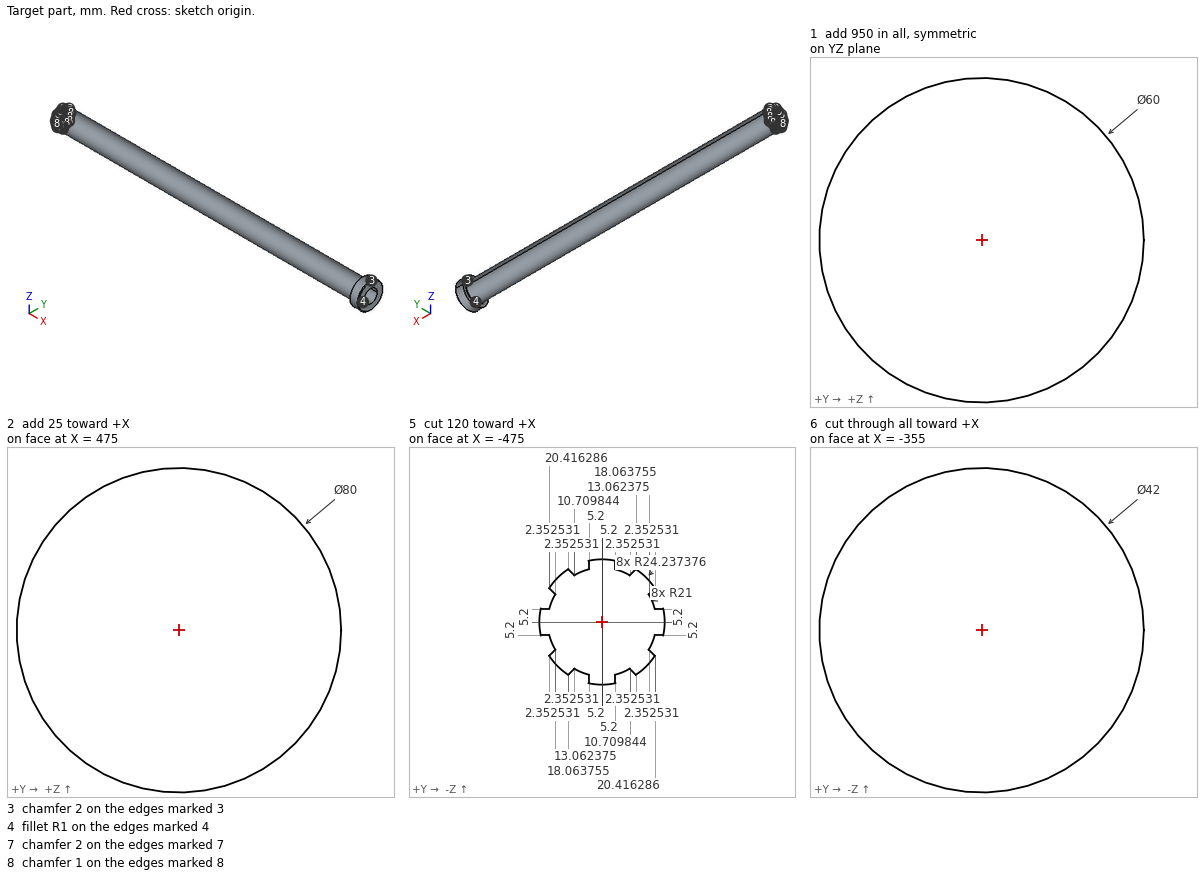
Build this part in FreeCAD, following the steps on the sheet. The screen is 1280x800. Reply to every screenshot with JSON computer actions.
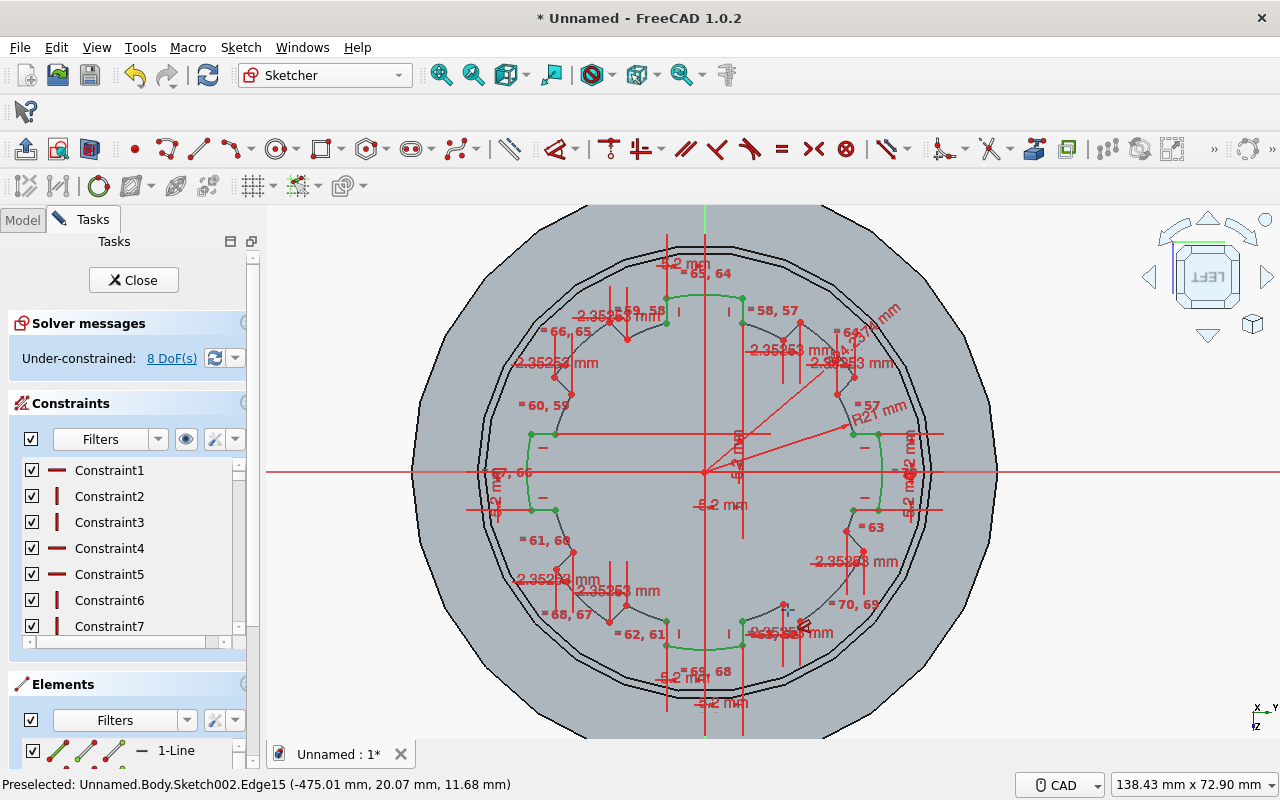
{"action": "left_click", "coordinate": [837, 395]}
{"action": "left_click", "coordinate": [802, 506]}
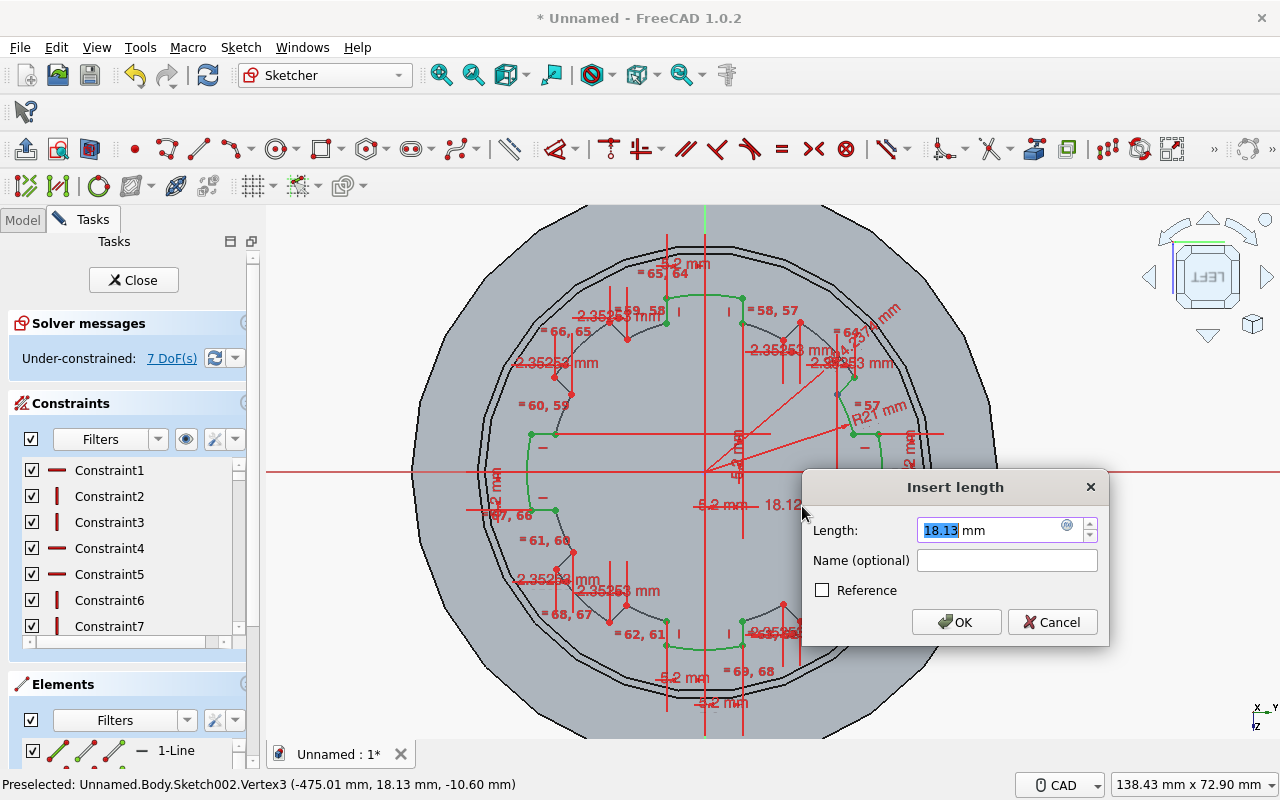
{"action": "type", "text": "18.063755"}
{"action": "key", "text": "Return"}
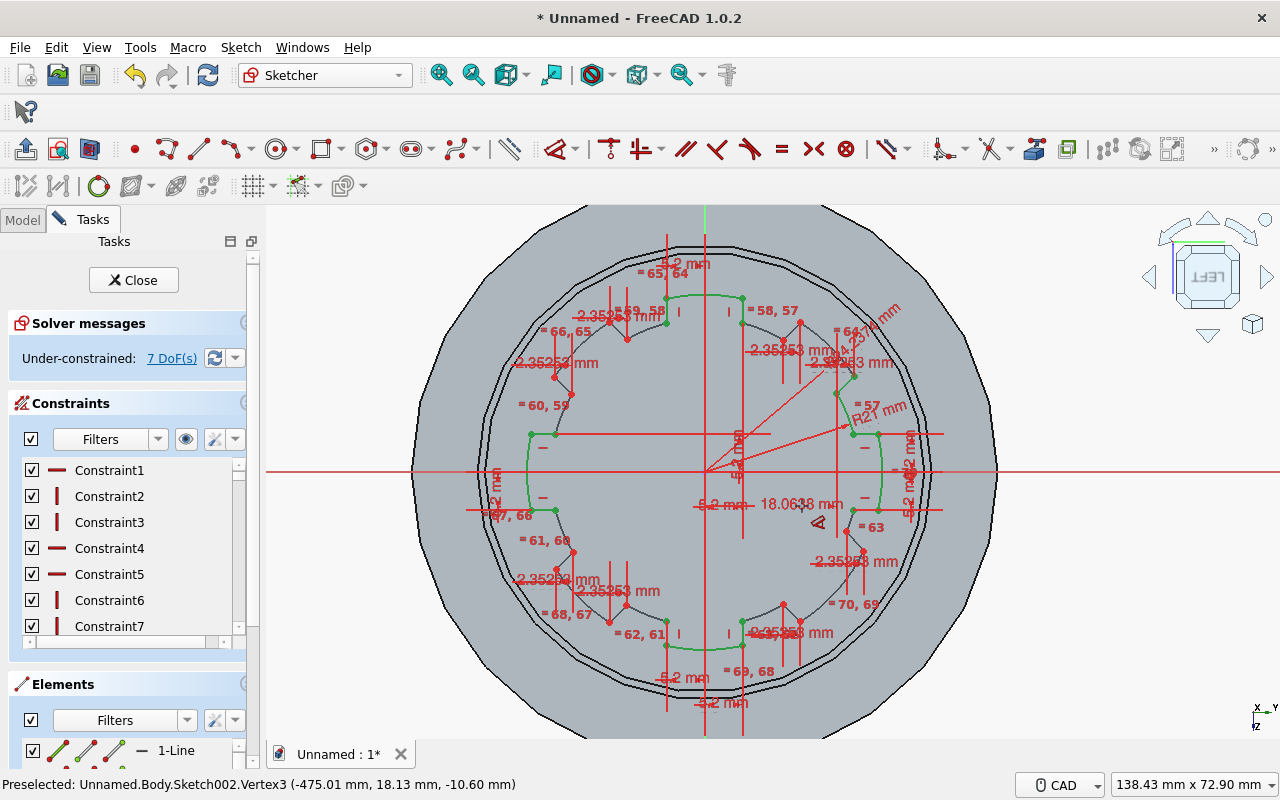
{"action": "left_click", "coordinate": [800, 323]}
{"action": "left_click", "coordinate": [753, 289]}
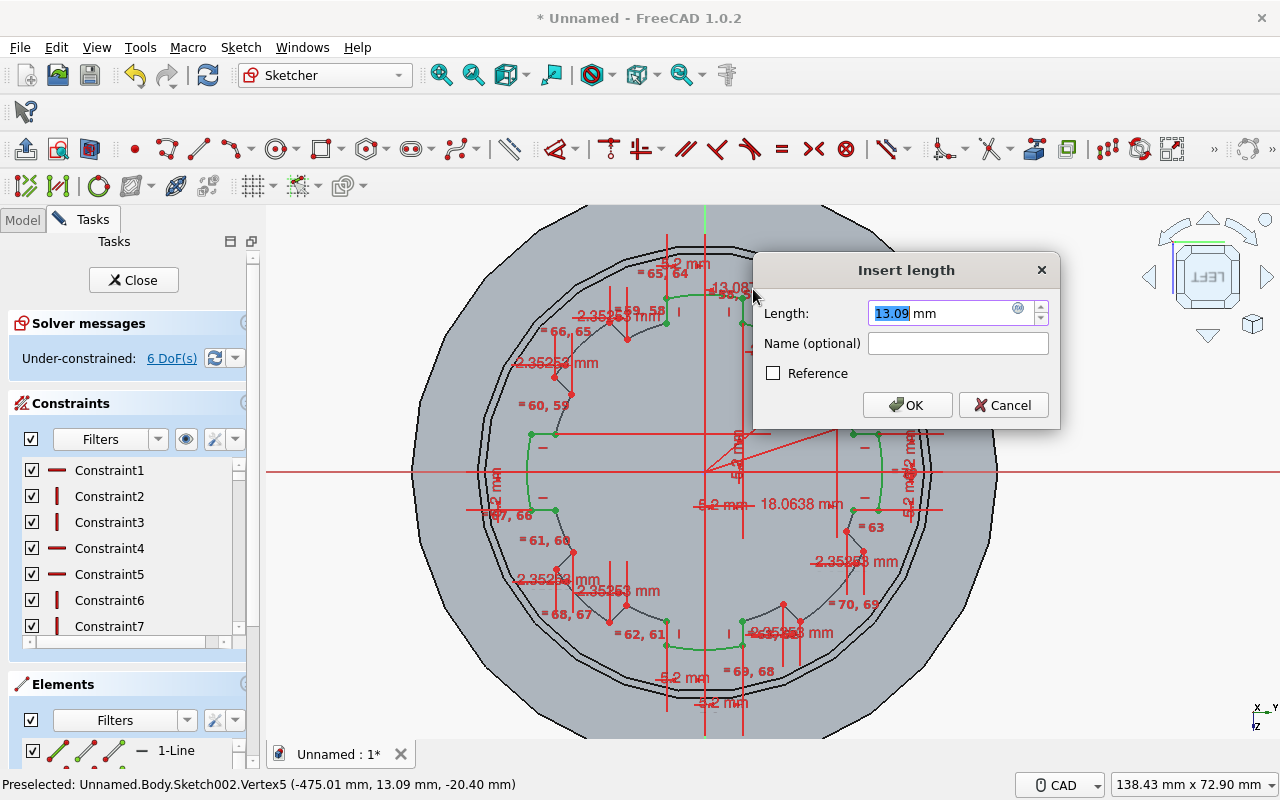
{"action": "type", "text": "13.062375"}
{"action": "key", "text": "Return"}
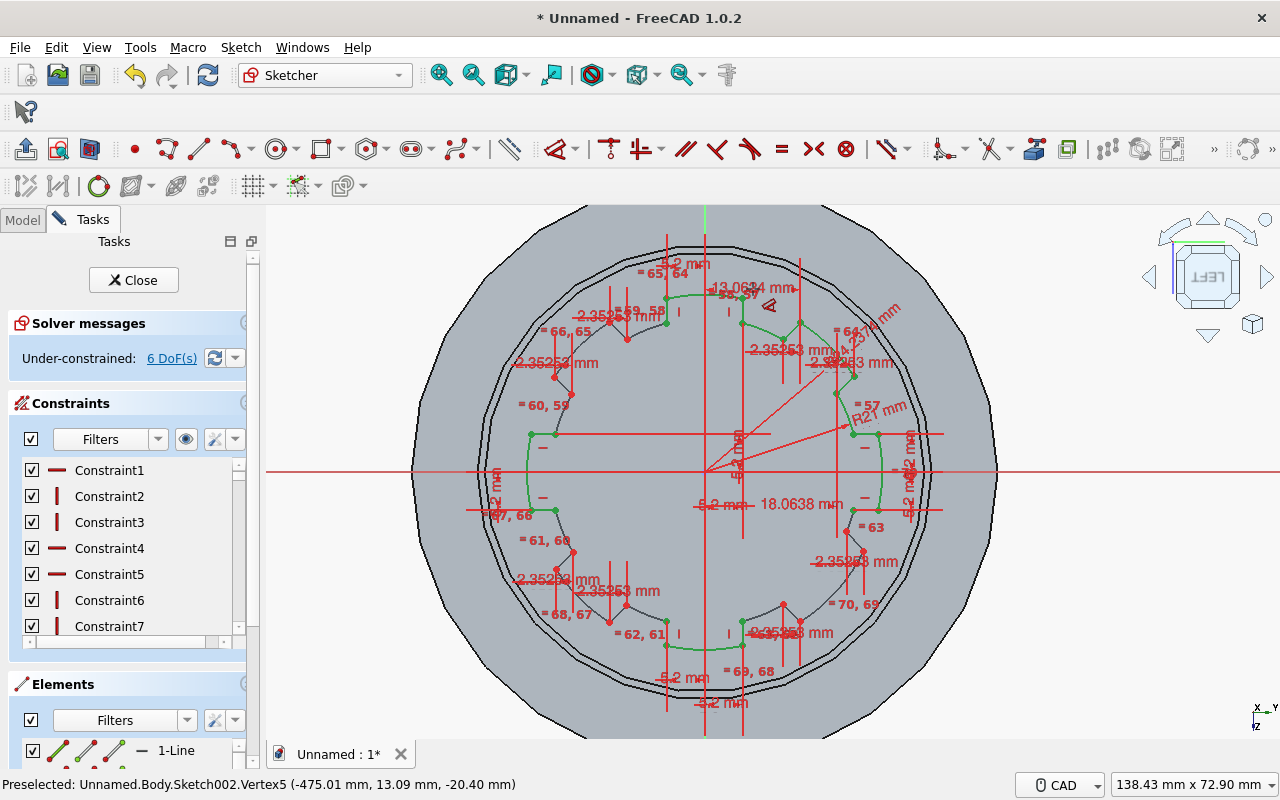
{"action": "left_click", "coordinate": [627, 339]}
{"action": "left_click", "coordinate": [648, 506]}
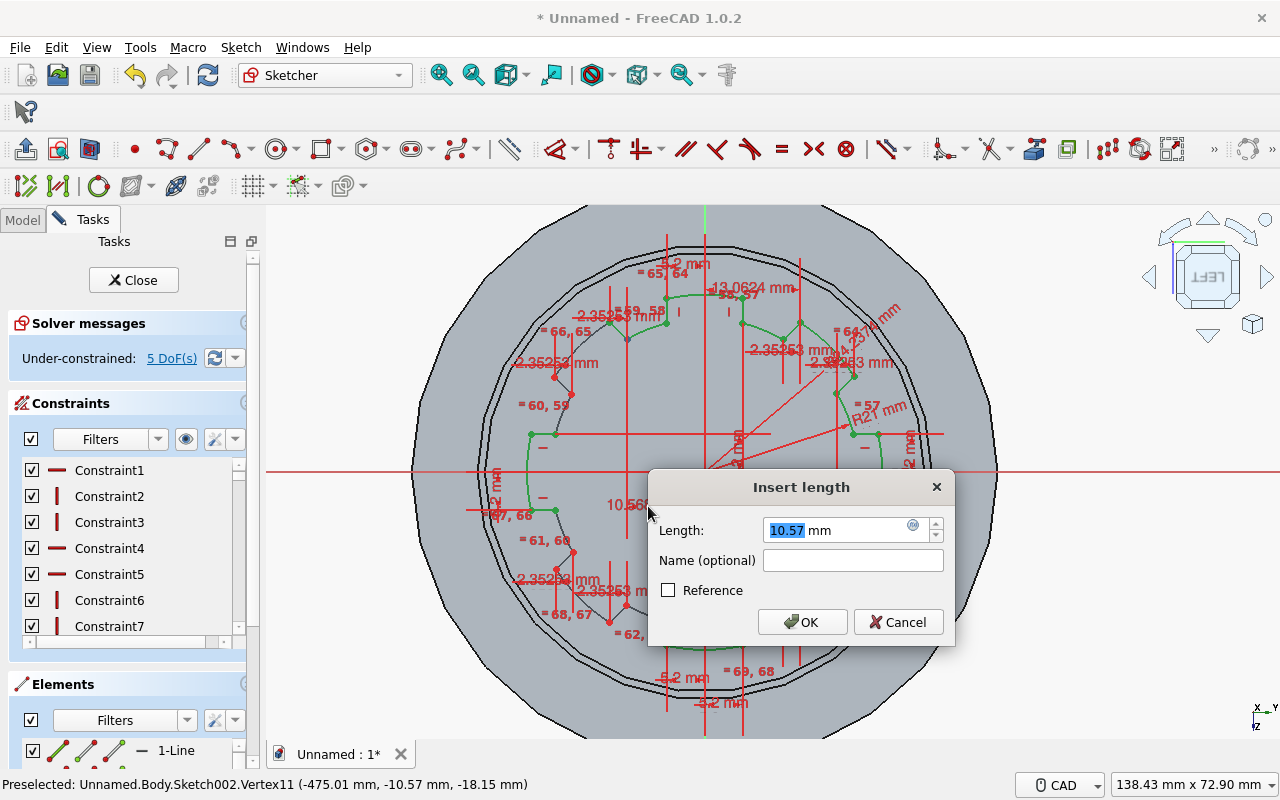
{"action": "type", "text": "10.709844"}
{"action": "key", "text": "Return"}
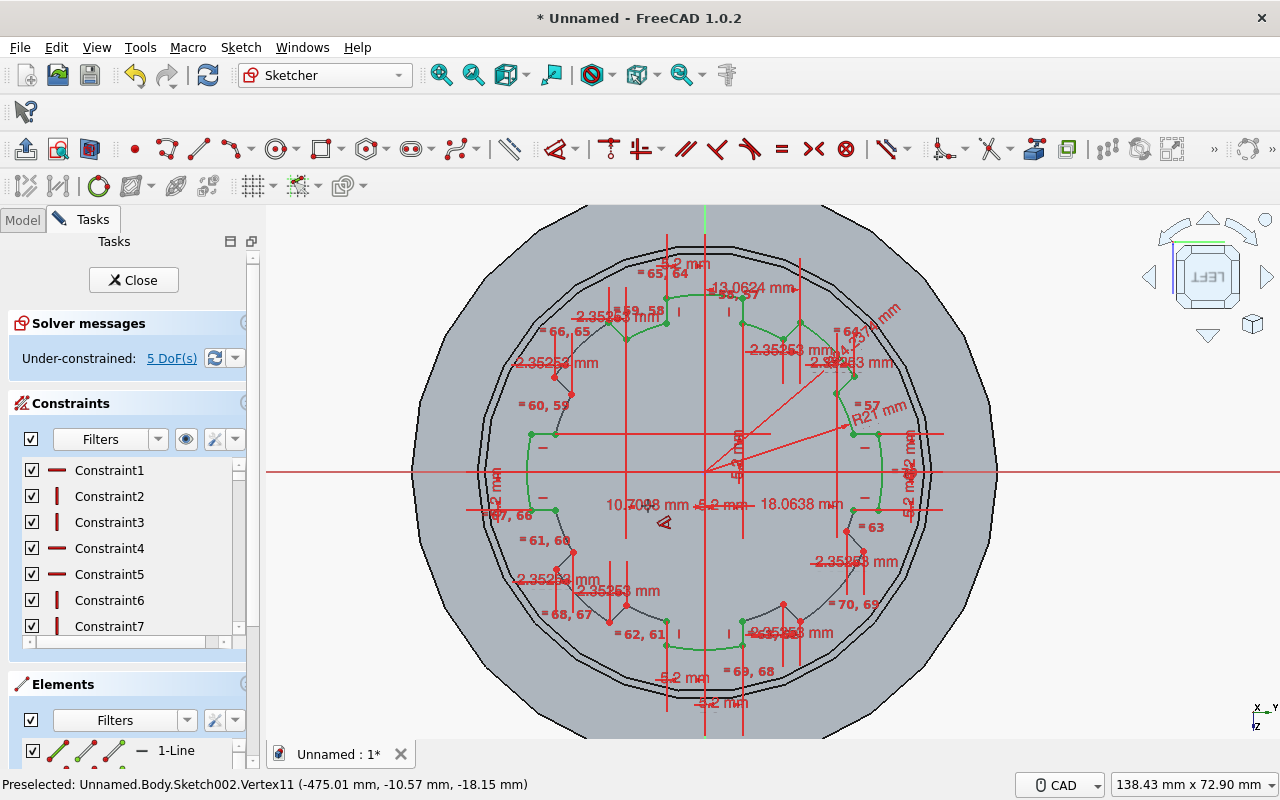
{"action": "left_click", "coordinate": [555, 377]}
{"action": "left_click", "coordinate": [664, 343]}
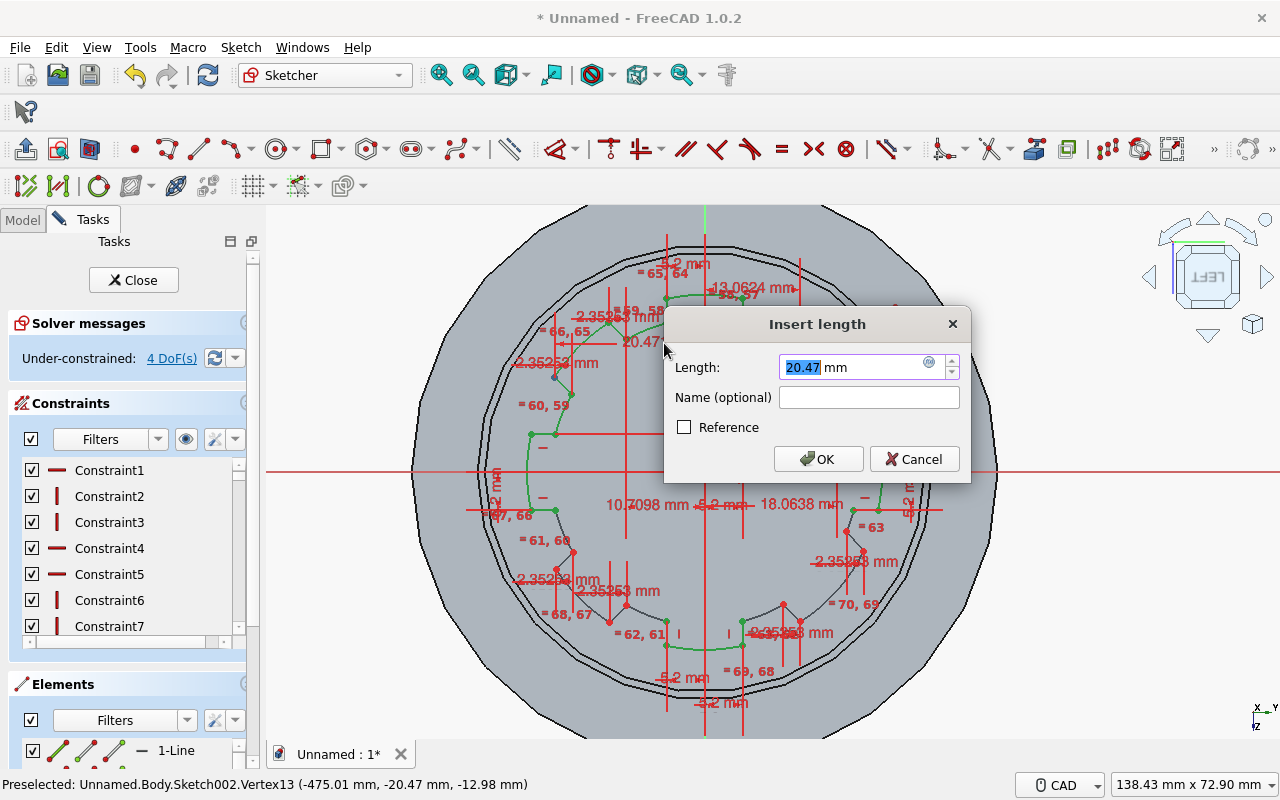
{"action": "type", "text": "20.416286"}
{"action": "key", "text": "Return"}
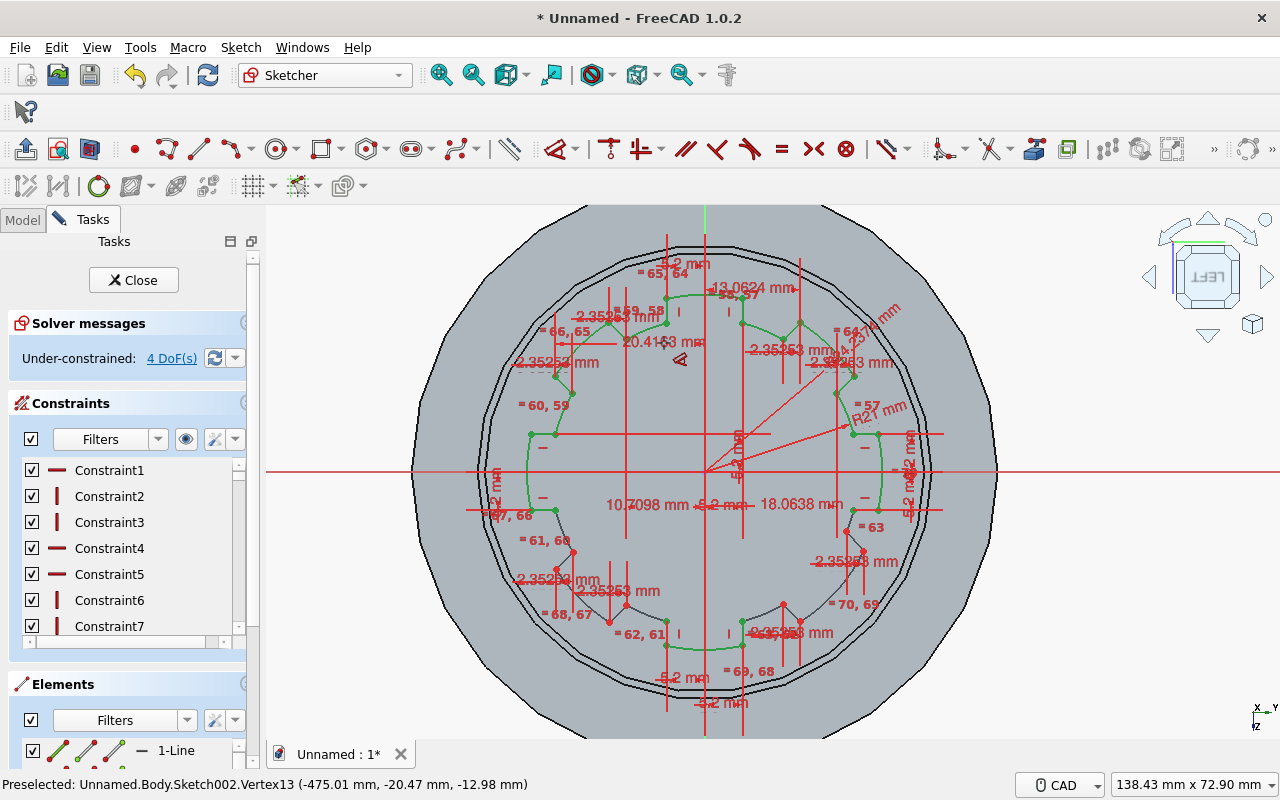
{"action": "left_click", "coordinate": [573, 552]}
{"action": "left_click", "coordinate": [639, 438]}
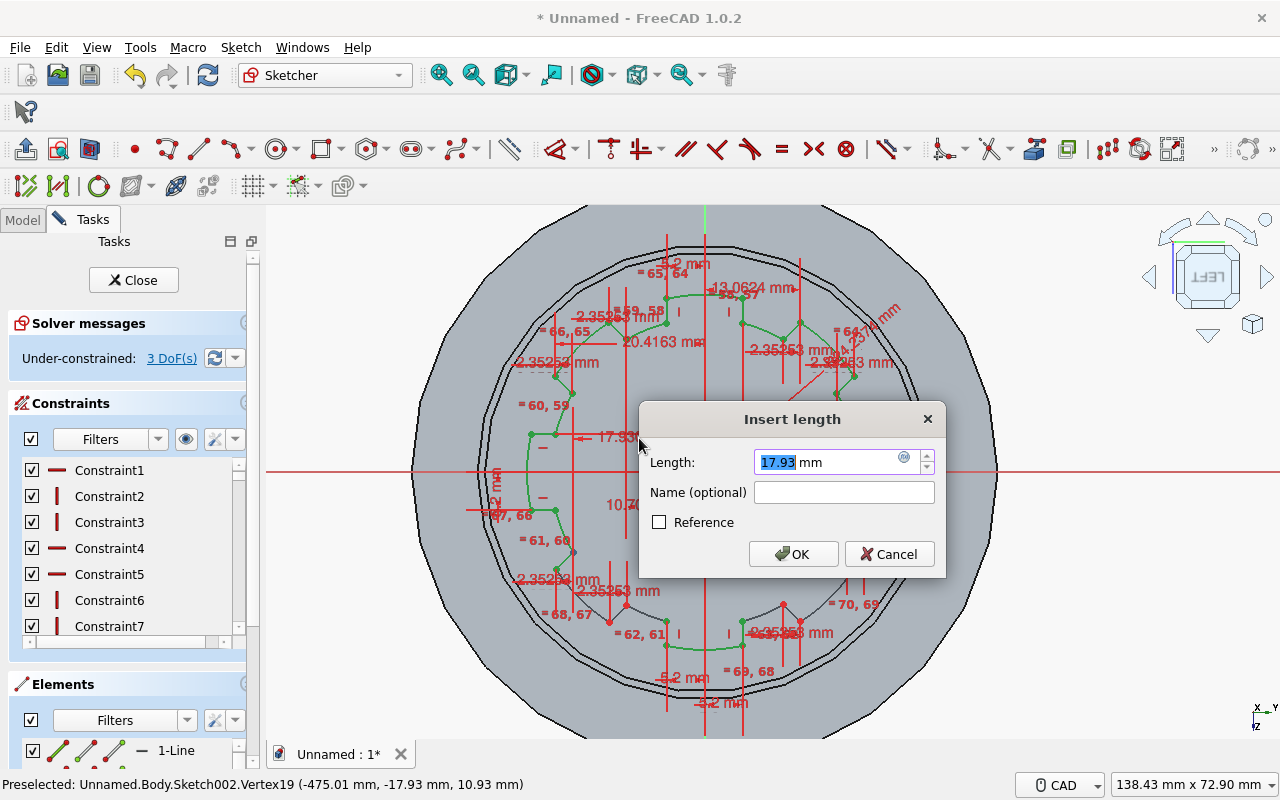
{"action": "type", "text": "18.063755"}
{"action": "key", "text": "Return"}